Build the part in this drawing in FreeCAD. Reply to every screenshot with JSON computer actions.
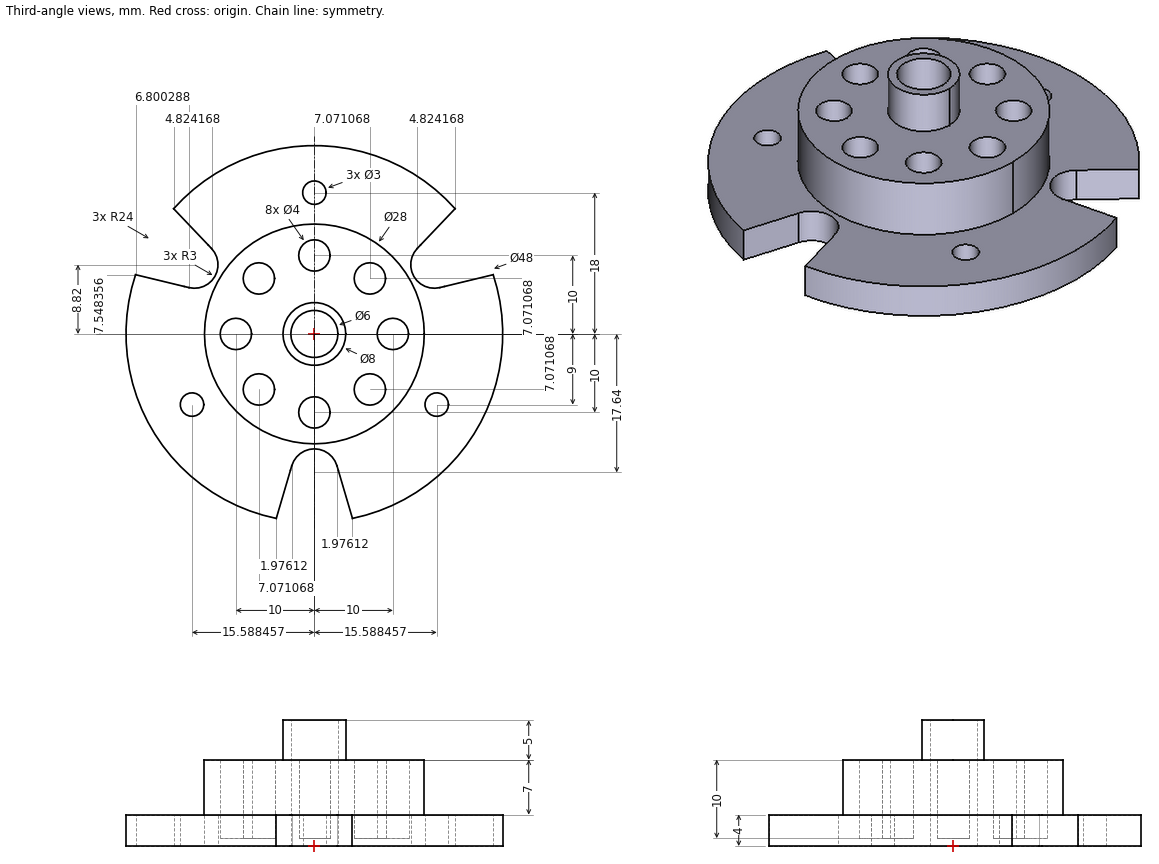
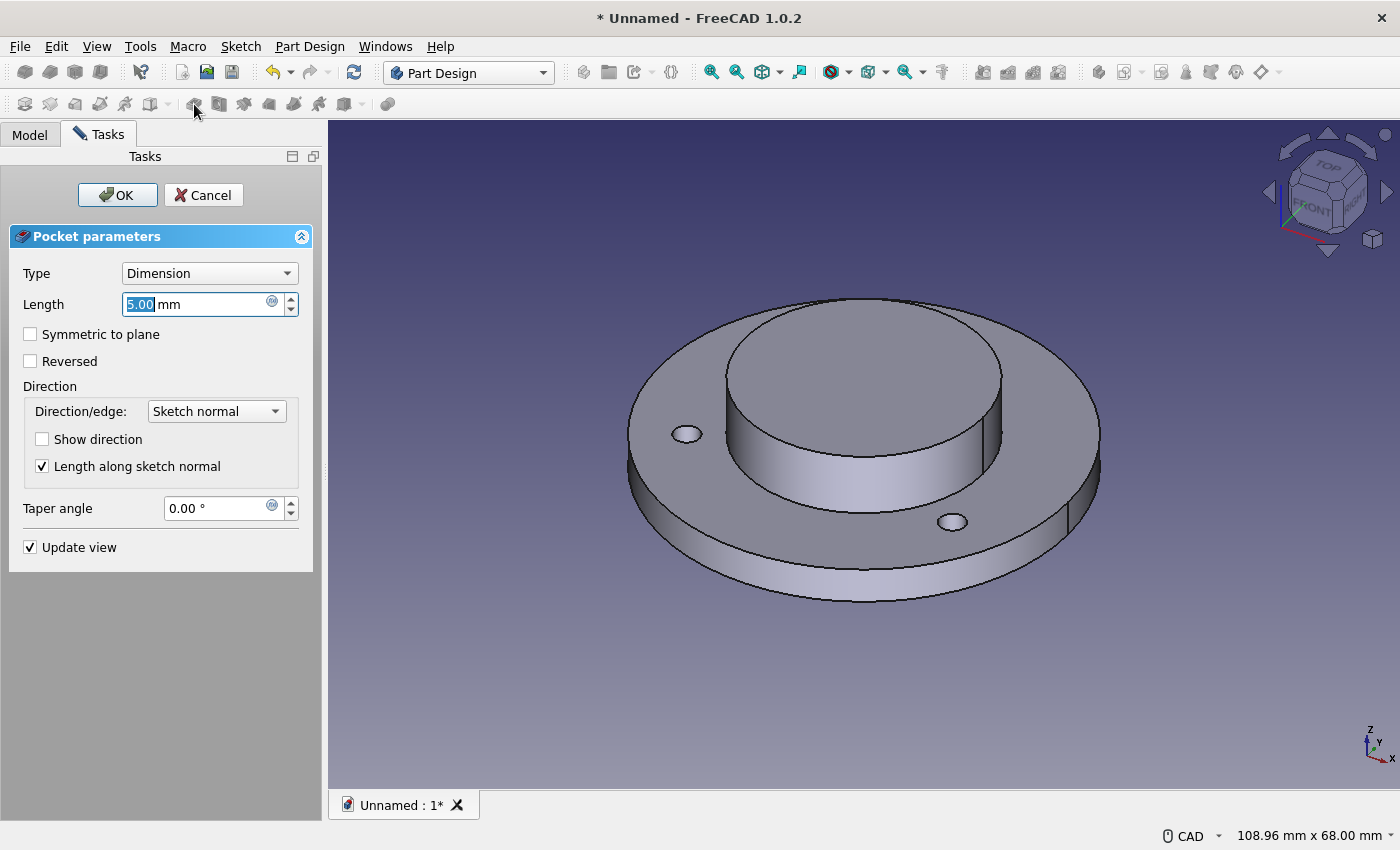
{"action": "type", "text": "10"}
{"action": "key", "text": "Tab"}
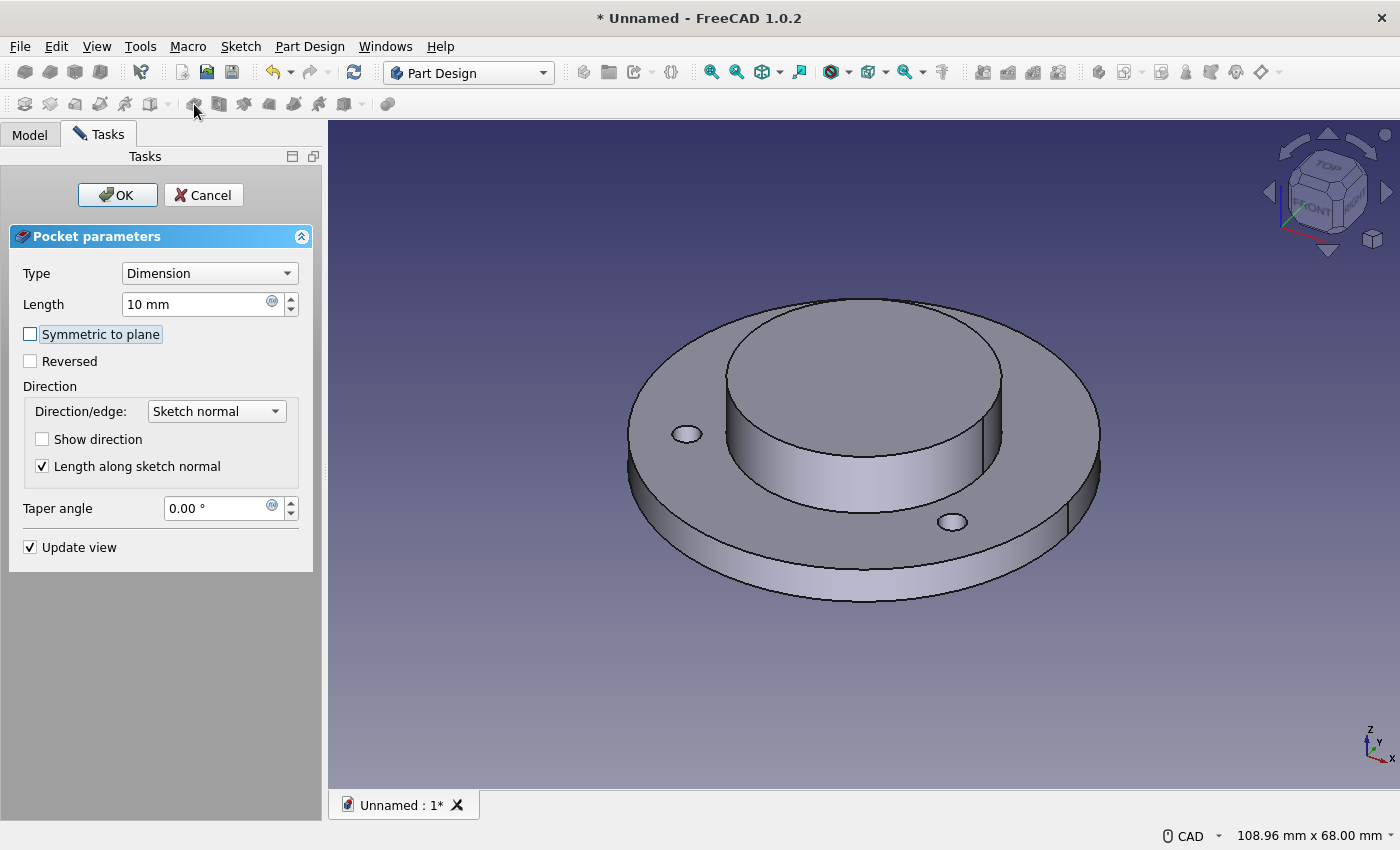
{"action": "left_click", "coordinate": [118, 195]}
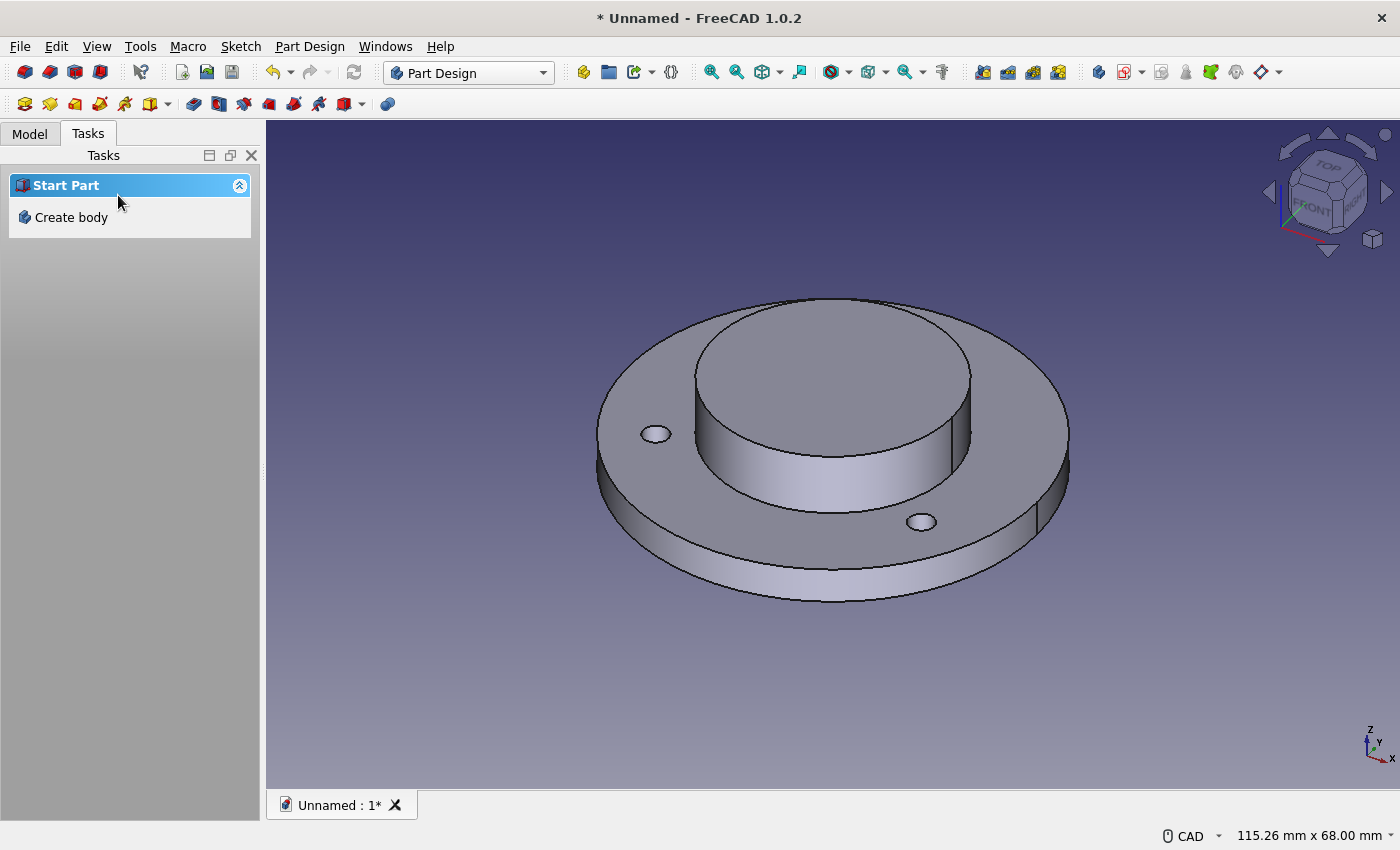
{"action": "left_click", "coordinate": [833, 377]}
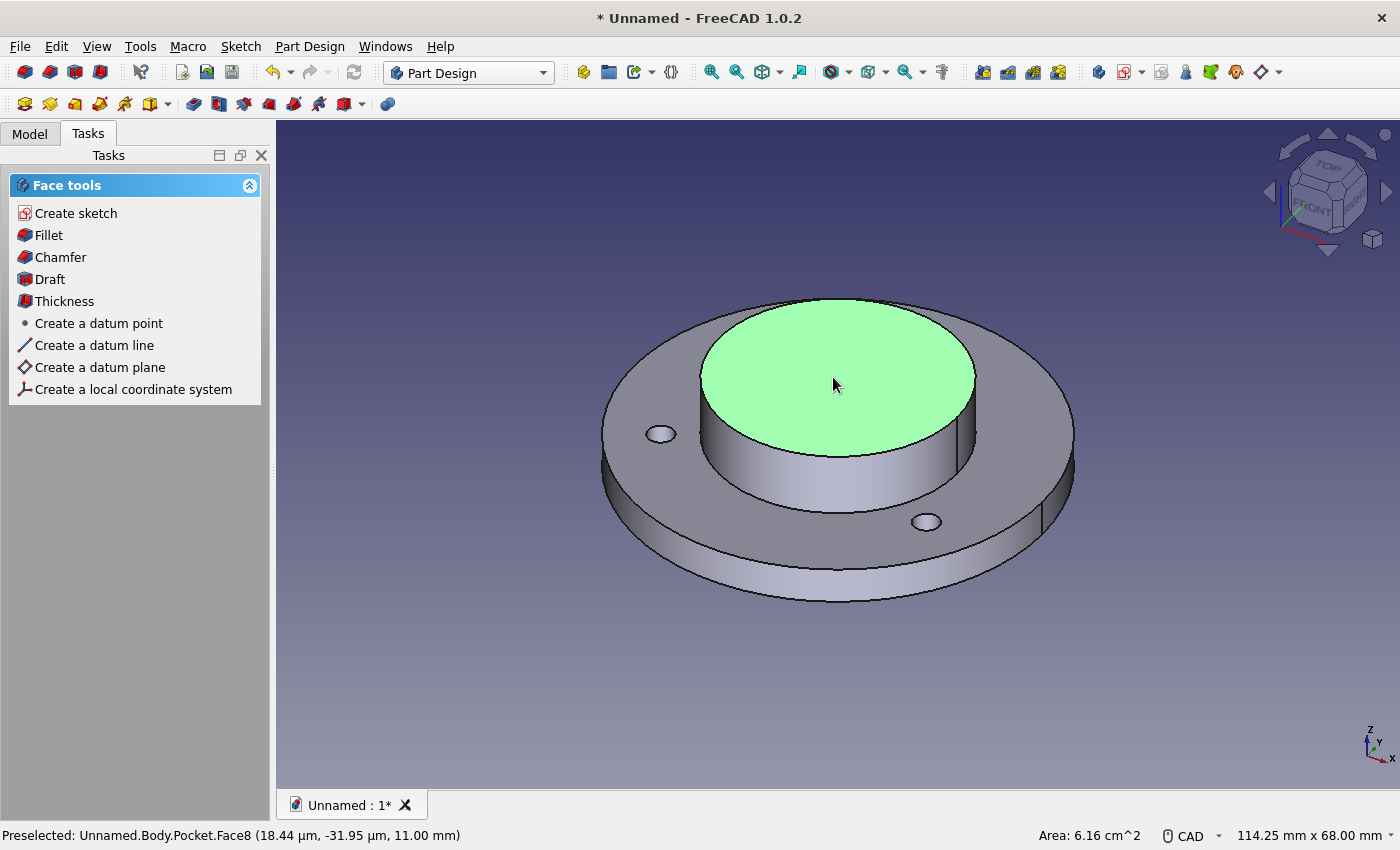
{"action": "left_click", "coordinate": [1124, 72]}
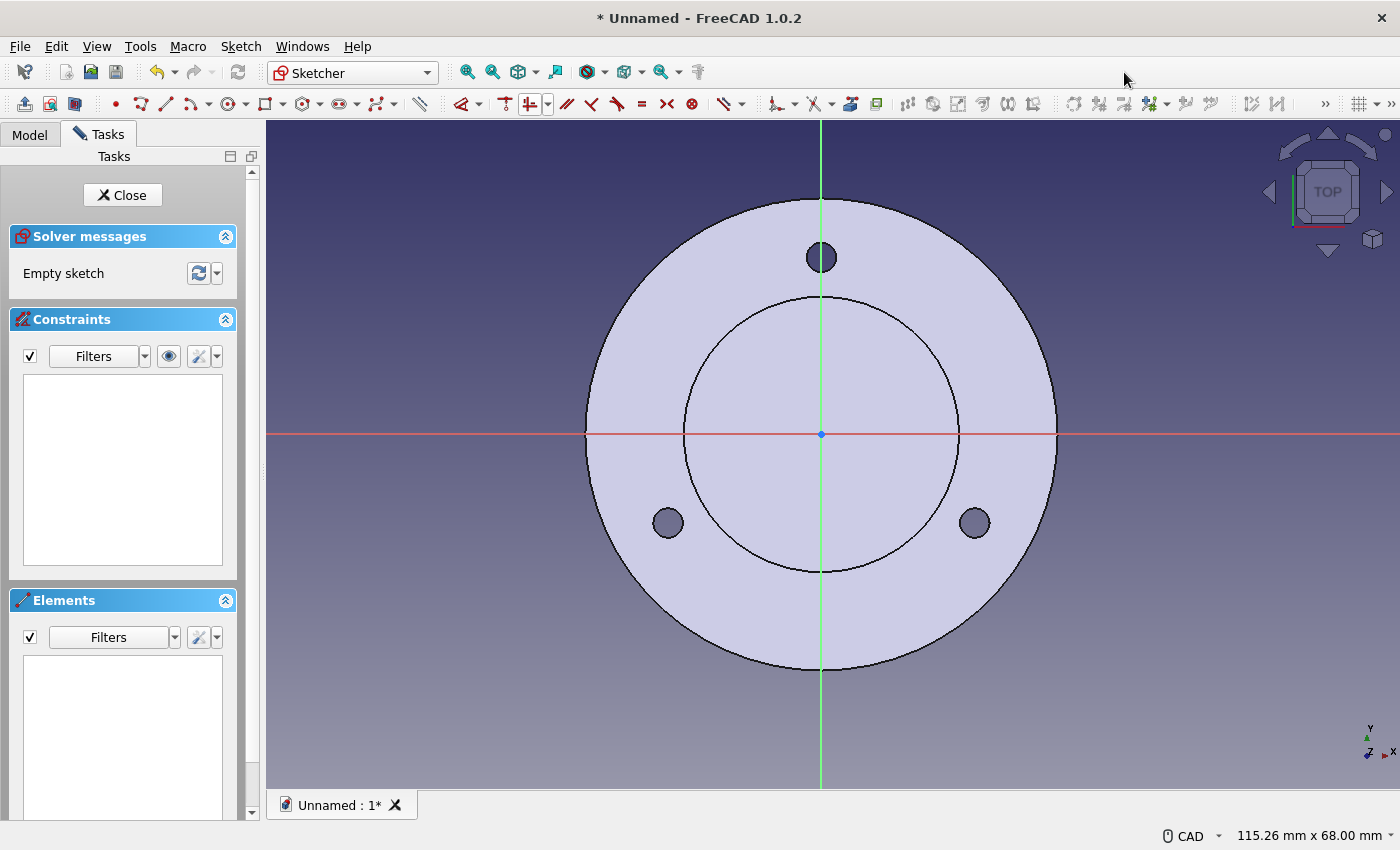
{"action": "scroll", "coordinate": [891, 410], "scroll_direction": "up", "scroll_amount": 3}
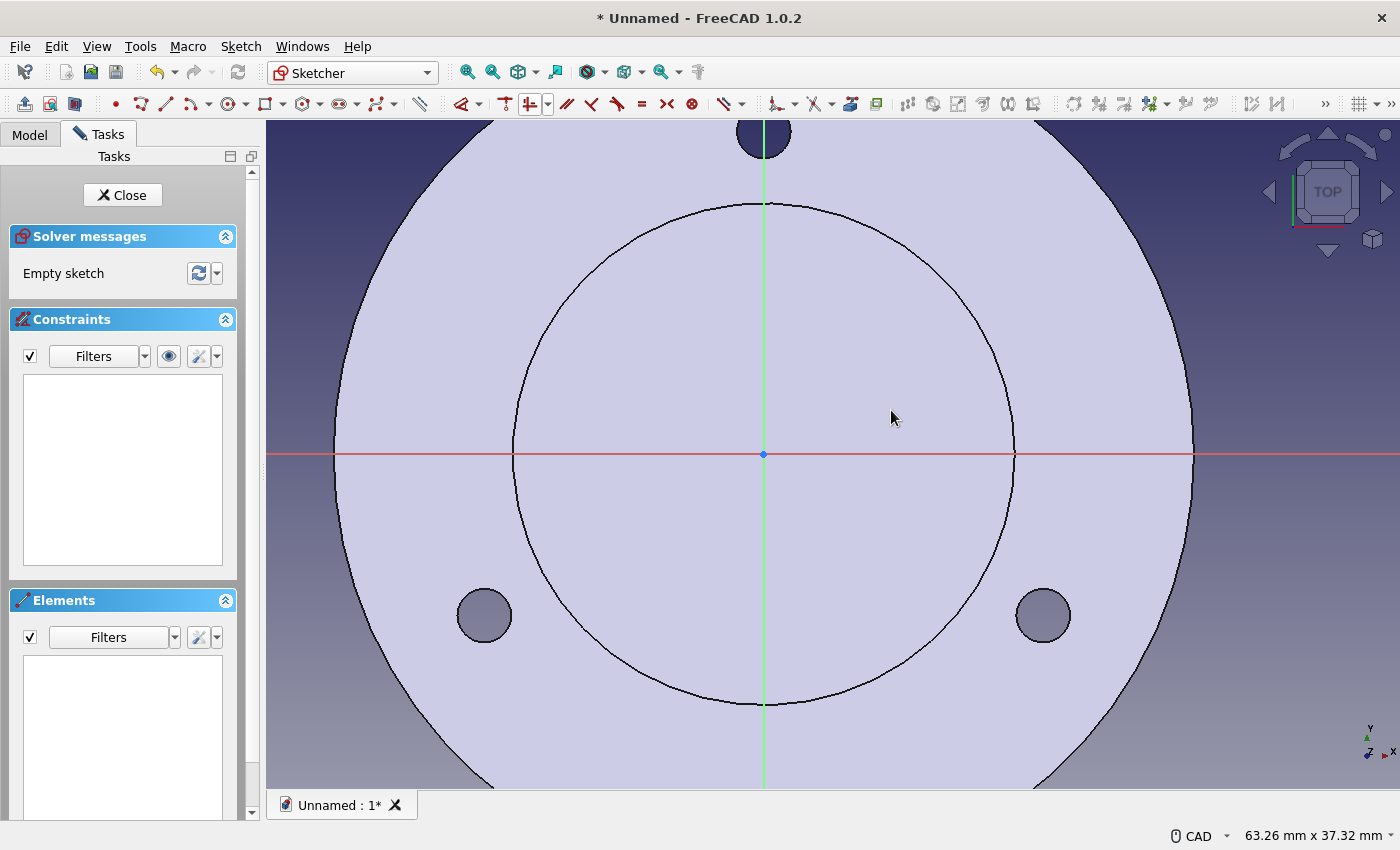
{"action": "key", "text": "g c"}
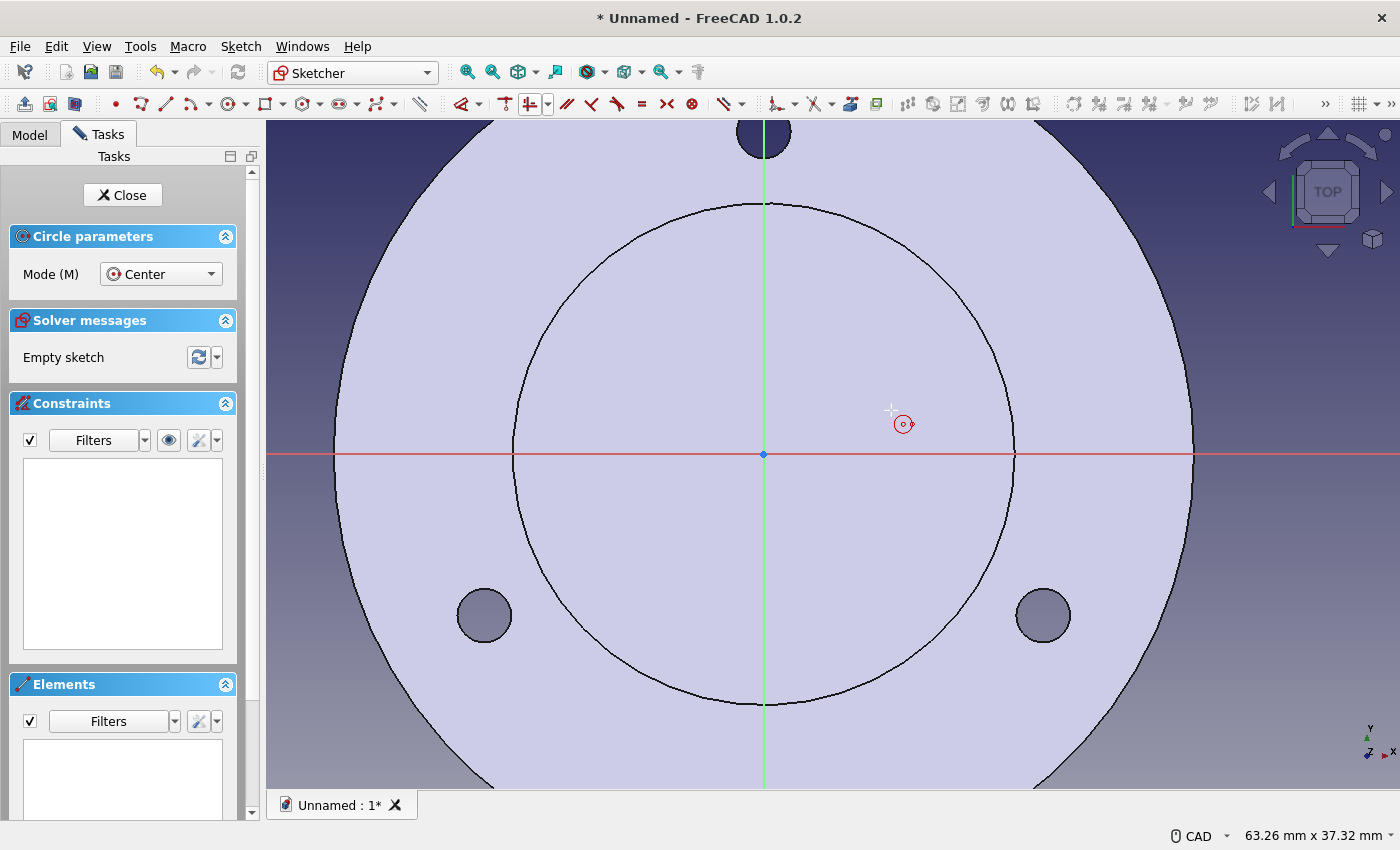
{"action": "left_click", "coordinate": [764, 275]}
{"action": "mouse_move", "coordinate": [789, 250]}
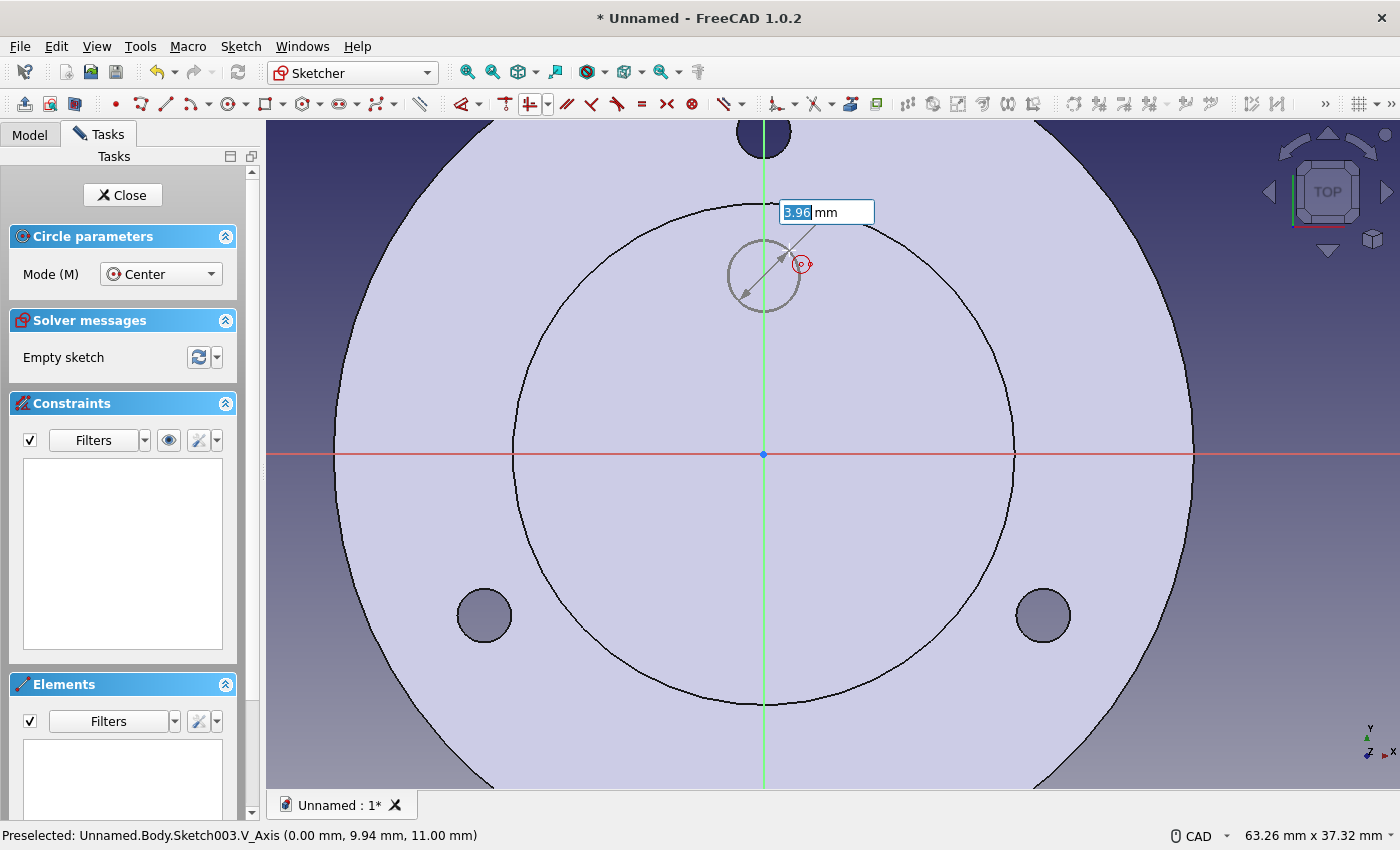
{"action": "type", "text": "4"}
{"action": "key", "text": "Return"}